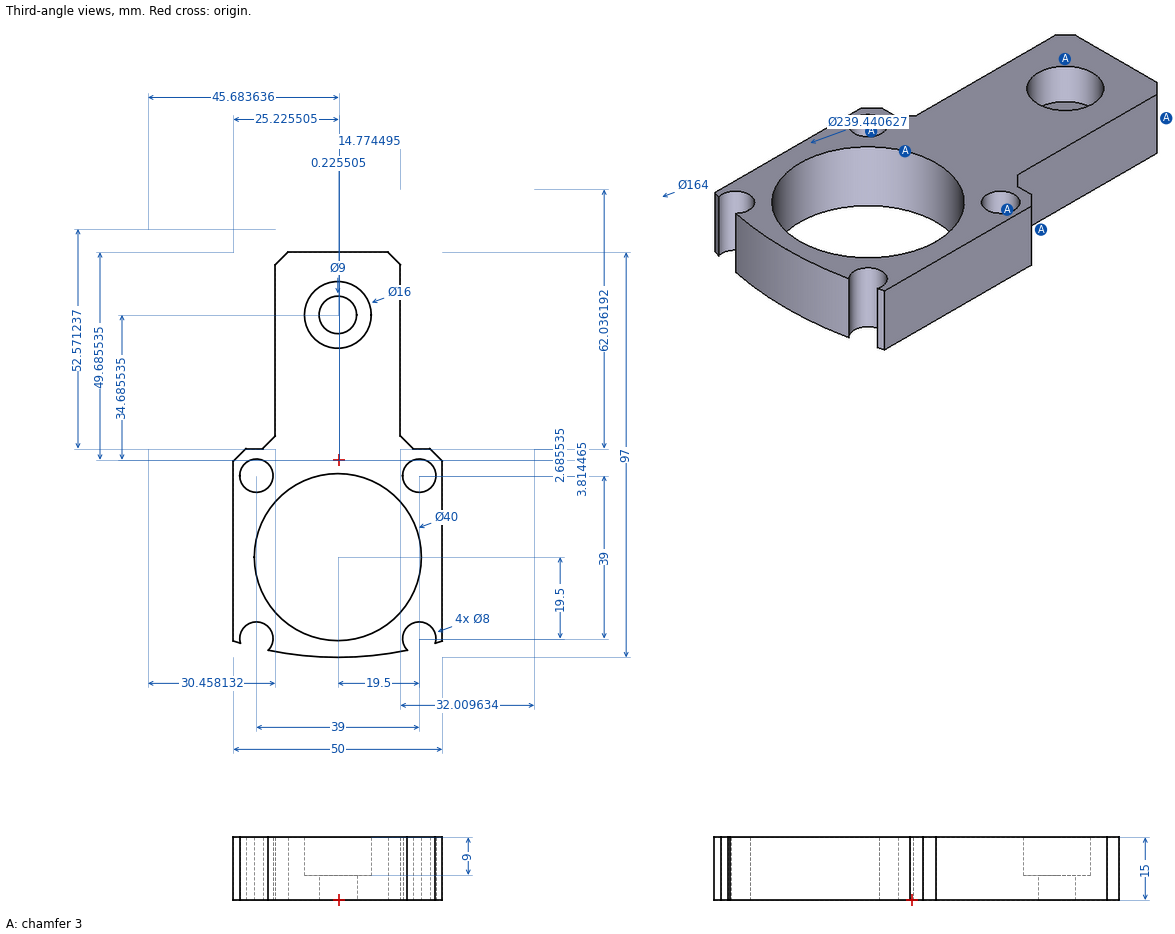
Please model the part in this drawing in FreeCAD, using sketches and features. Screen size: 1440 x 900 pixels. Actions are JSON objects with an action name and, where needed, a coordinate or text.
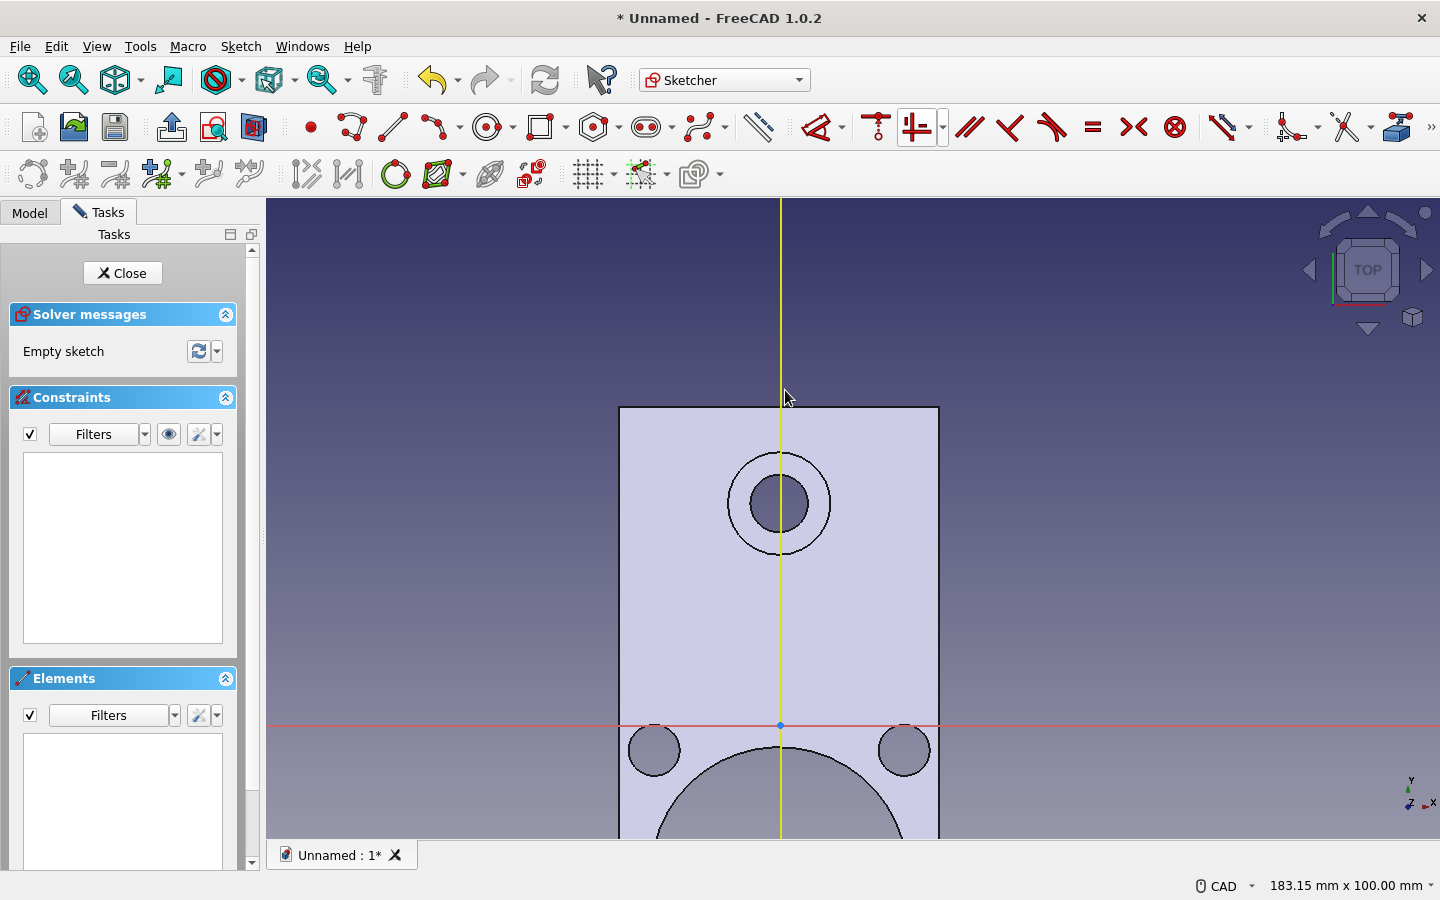
{"action": "left_click", "coordinate": [540, 128]}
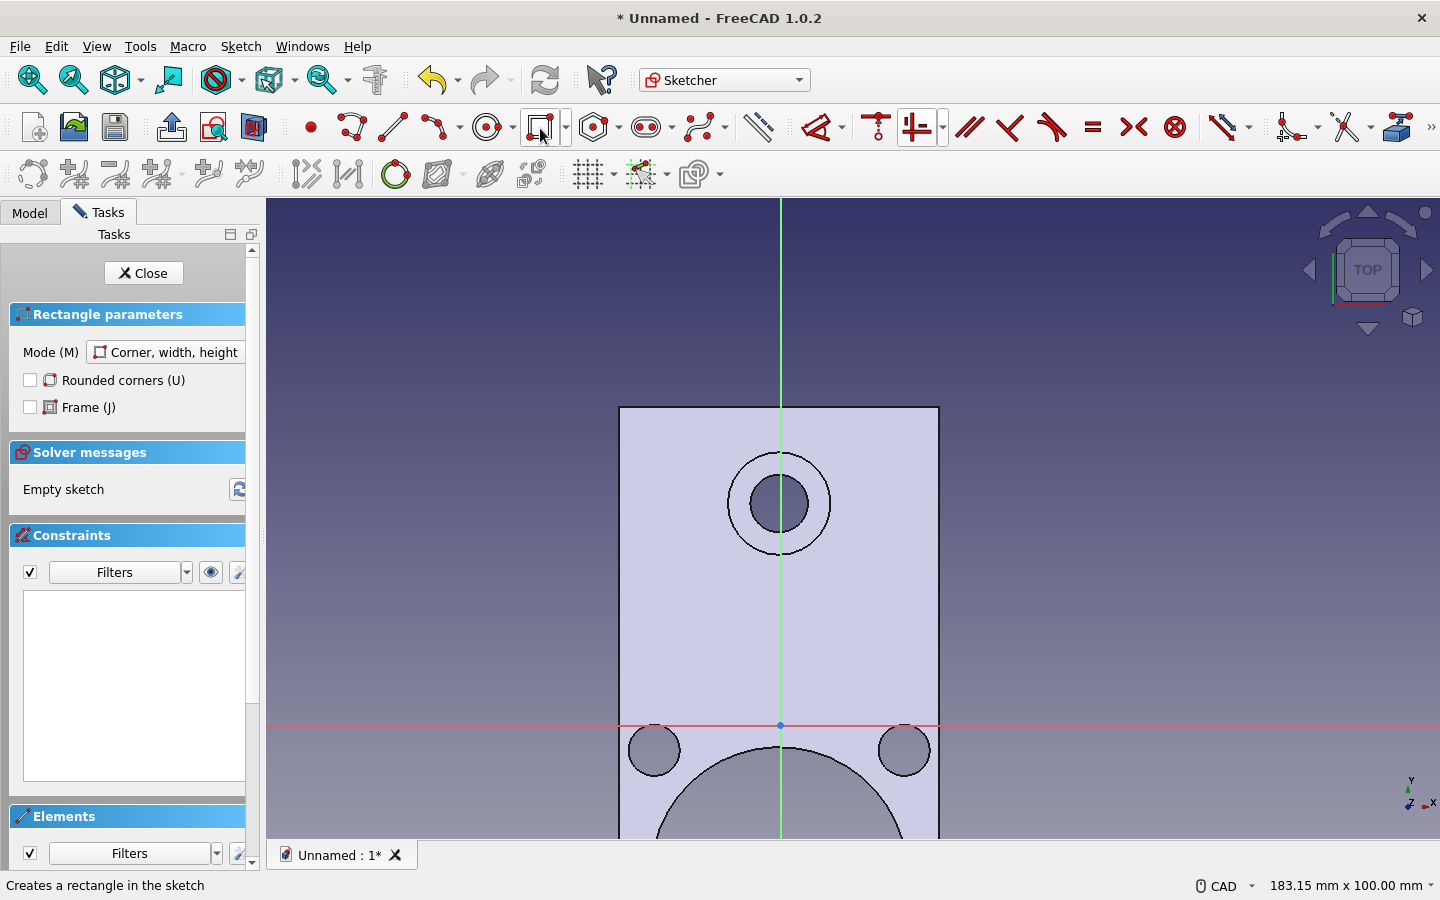
{"action": "left_click", "coordinate": [875, 311]}
{"action": "mouse_move", "coordinate": [1081, 709]}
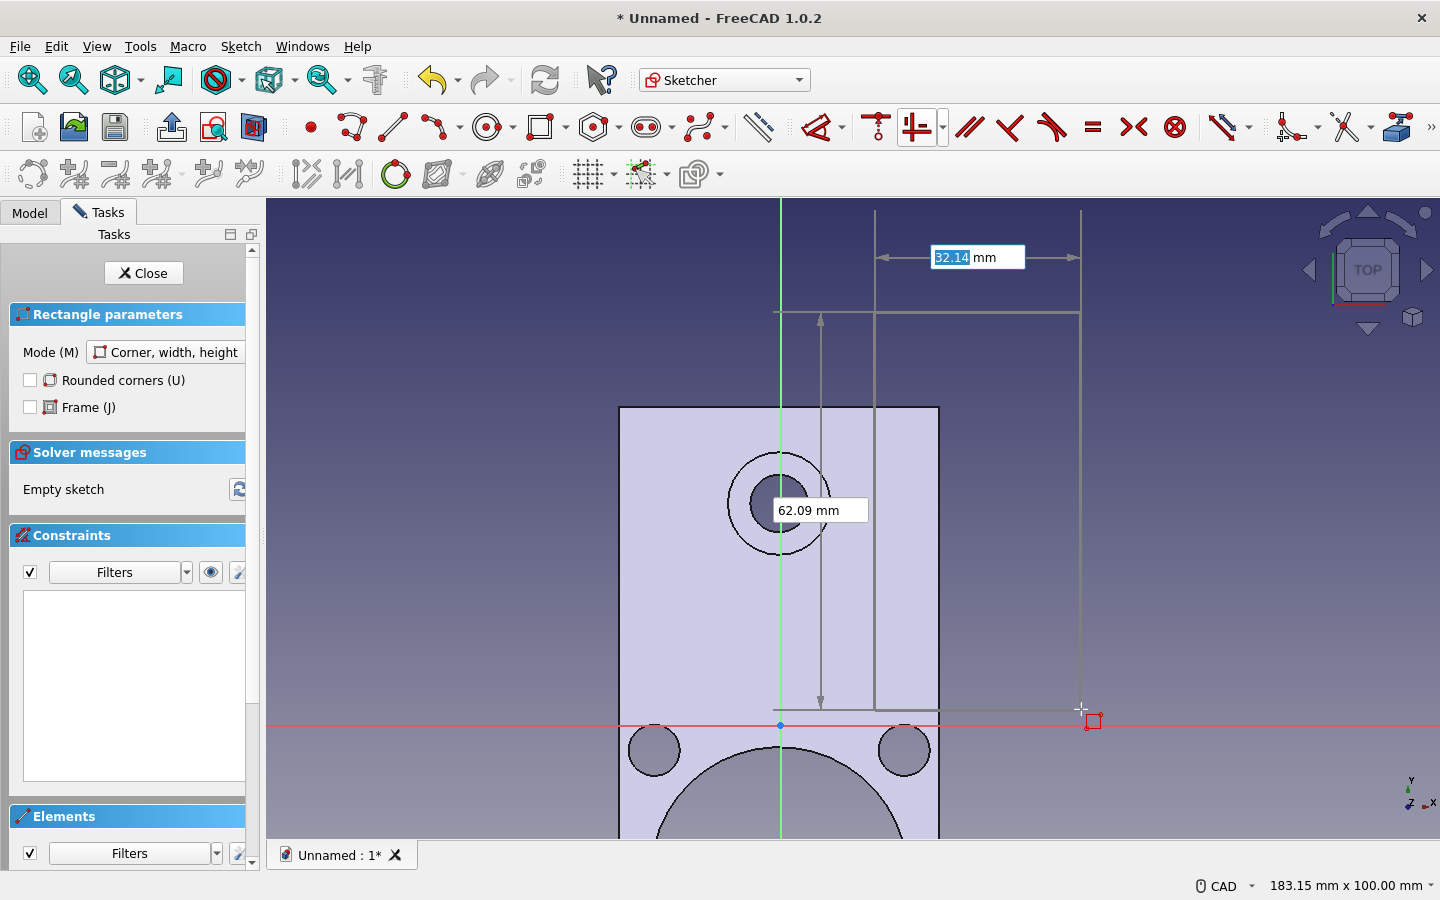
{"action": "type", "text": "32.009634"}
{"action": "key", "text": "Tab"}
{"action": "type", "text": "62.036192"}
{"action": "key", "text": "Return"}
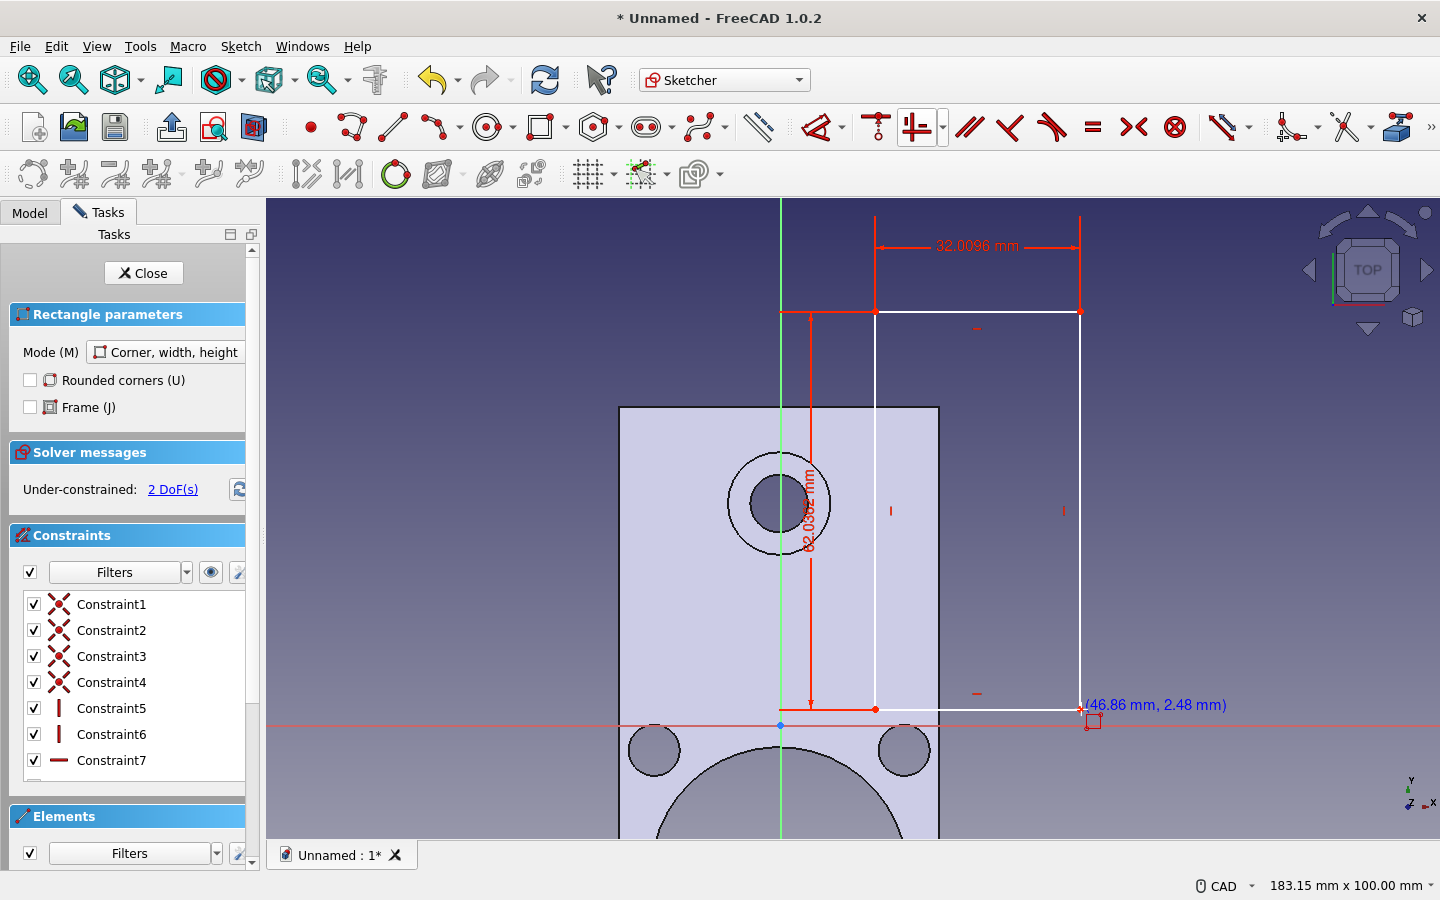
{"action": "left_click", "coordinate": [488, 372]}
{"action": "mouse_move", "coordinate": [683, 709]}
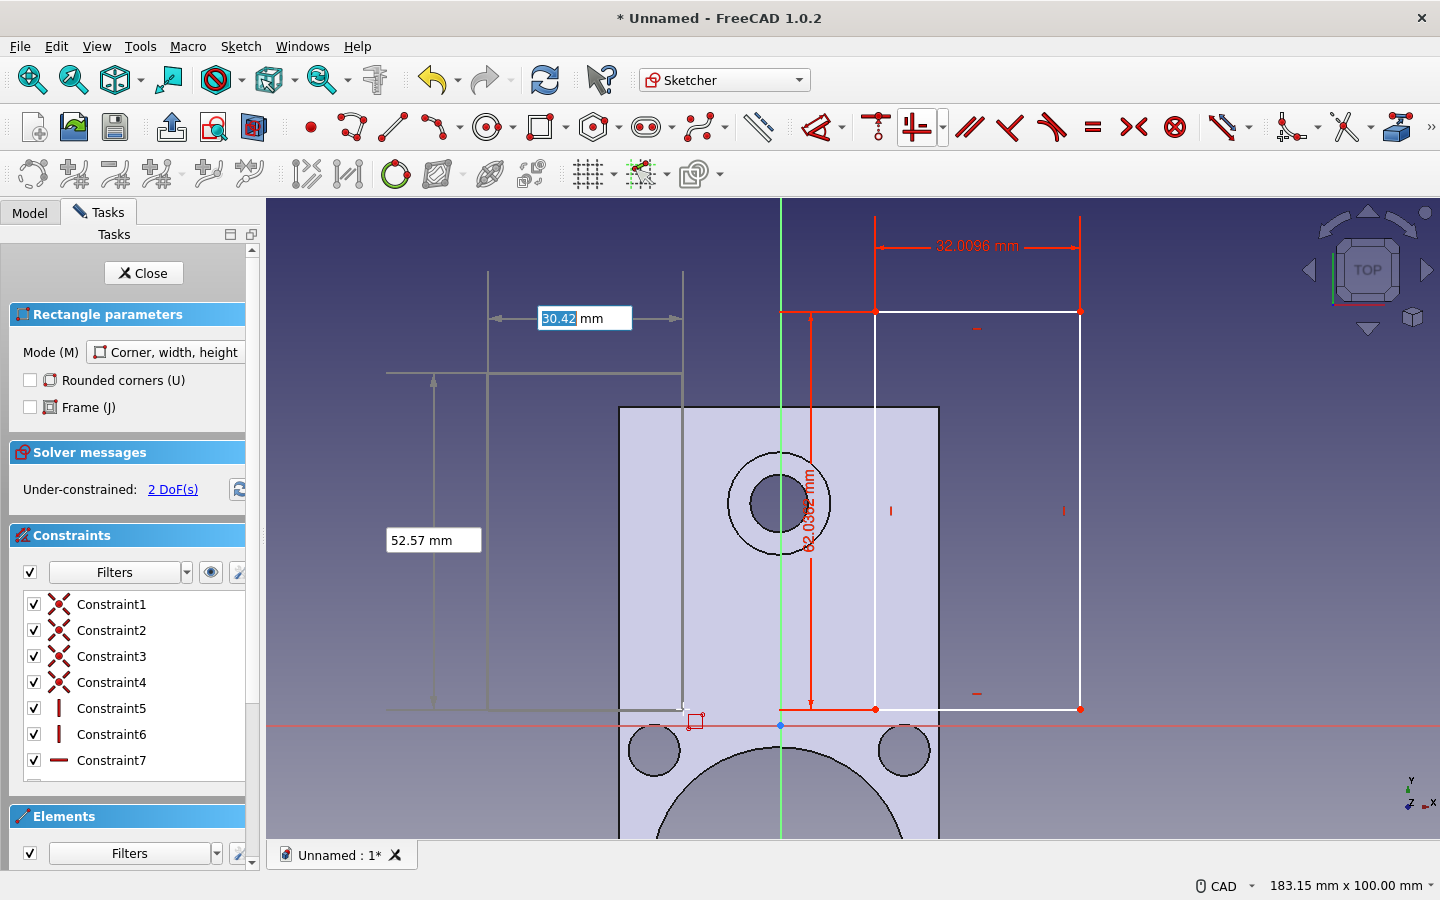
{"action": "type", "text": "30.458132"}
{"action": "key", "text": "Tab"}
{"action": "type", "text": "52.571237"}
{"action": "key", "text": "Return"}
{"action": "key", "text": "Escape"}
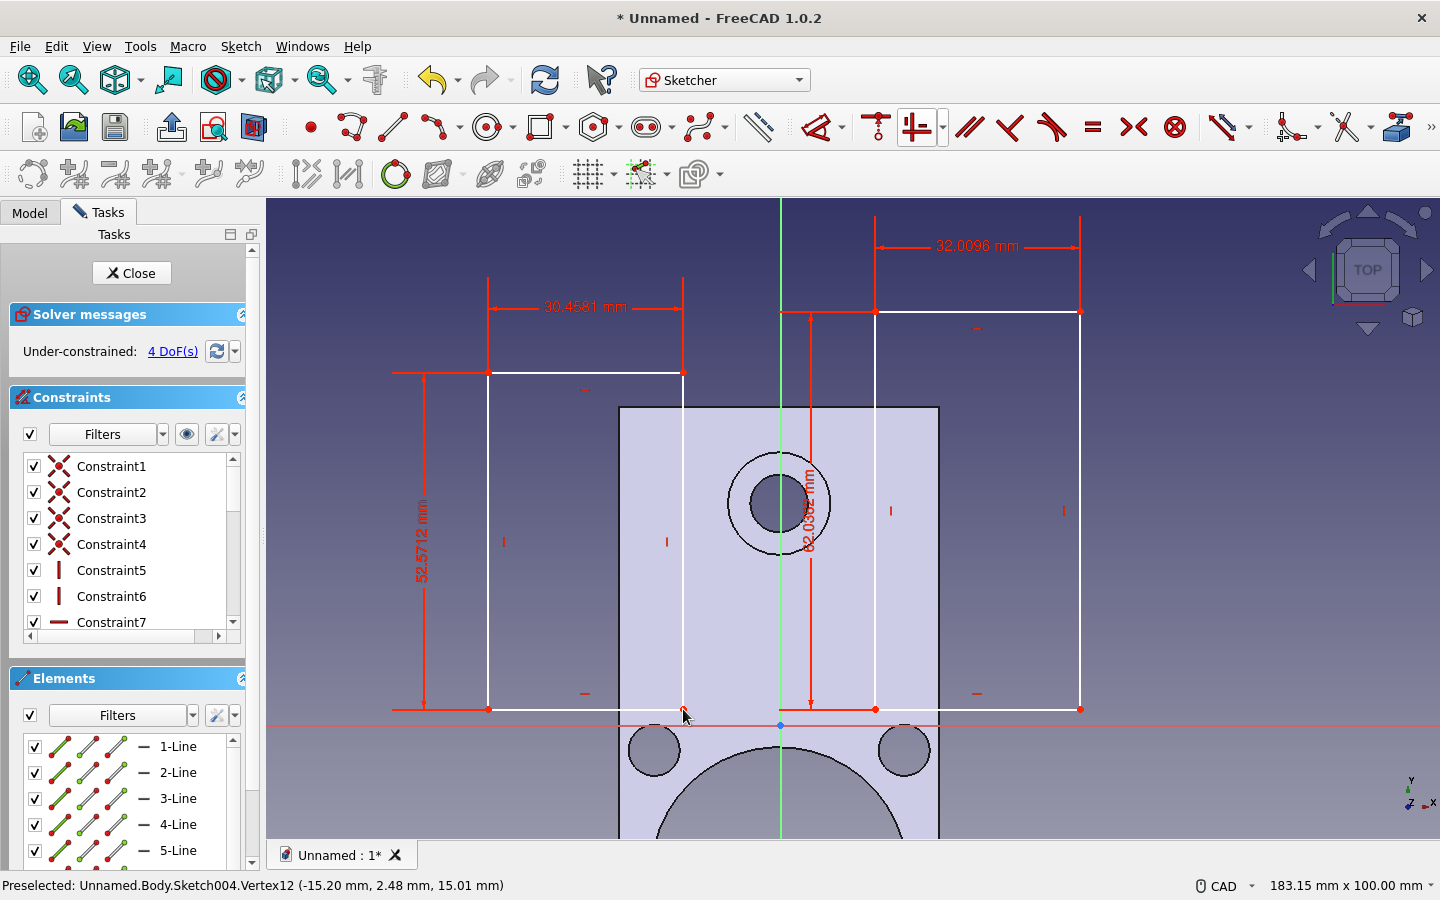
{"action": "key", "text": "d"}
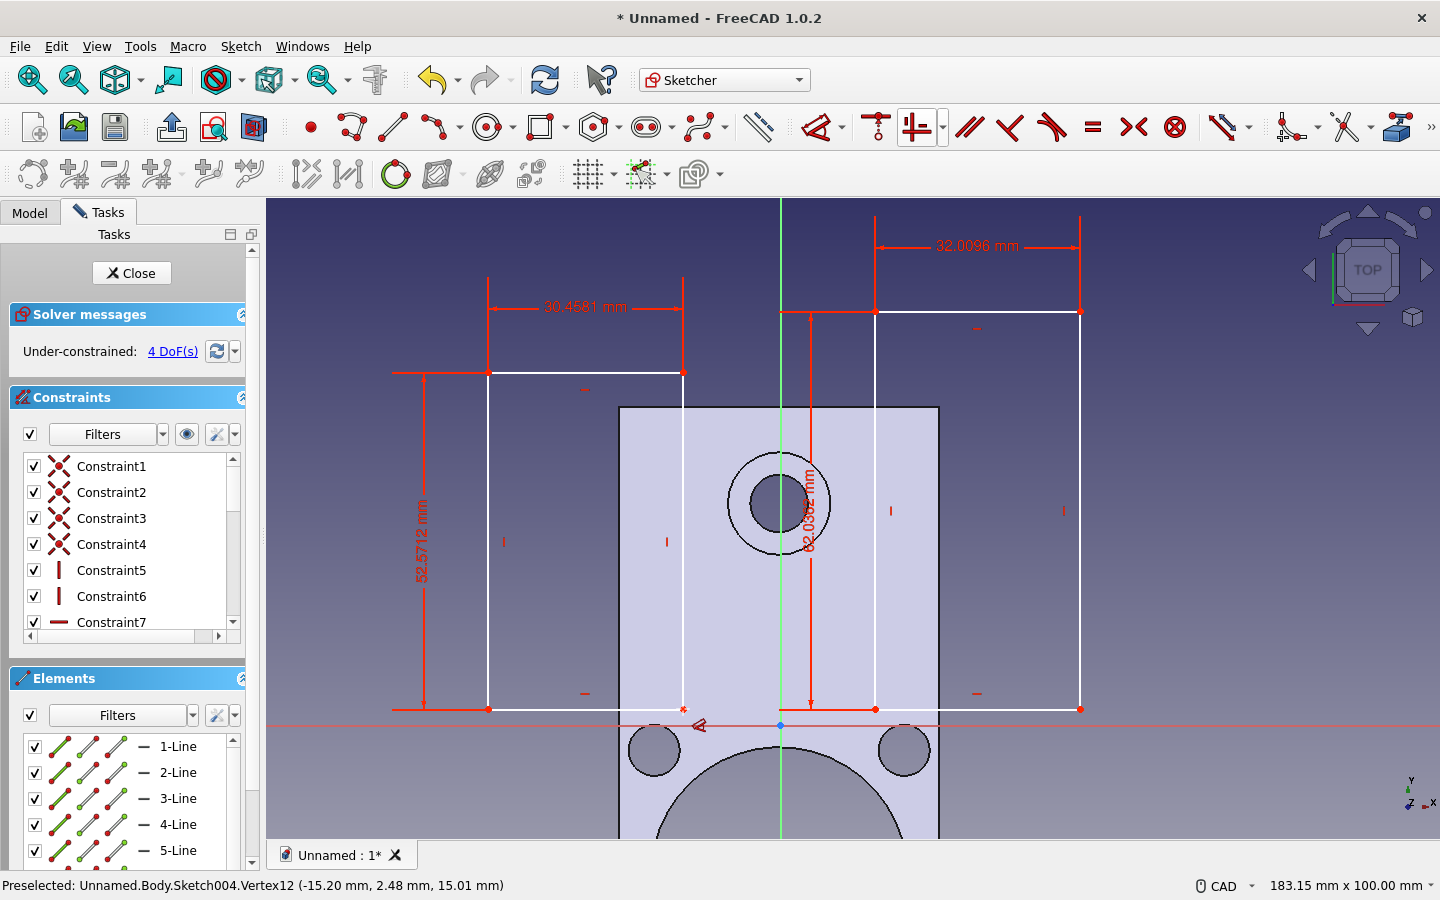
{"action": "scroll", "coordinate": [875, 710], "scroll_direction": "up", "scroll_amount": 5}